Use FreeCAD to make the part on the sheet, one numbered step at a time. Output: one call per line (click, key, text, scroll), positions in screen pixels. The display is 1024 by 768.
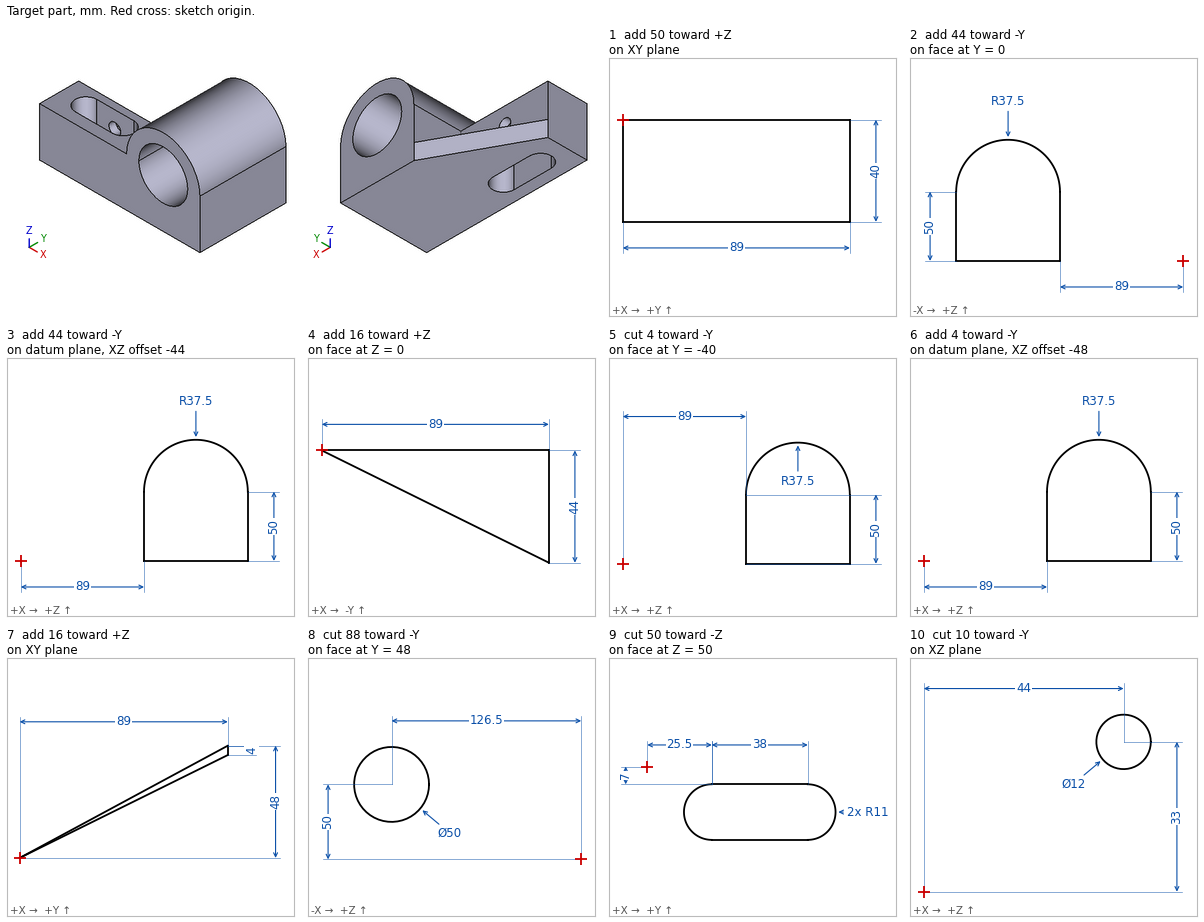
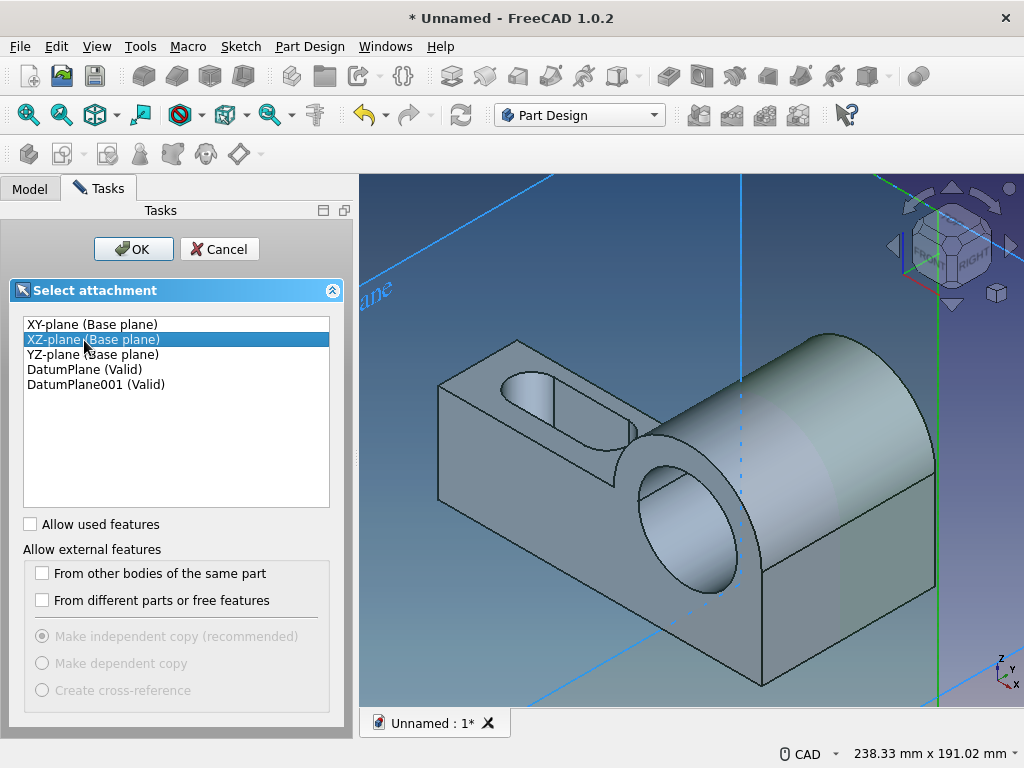
click(134, 249)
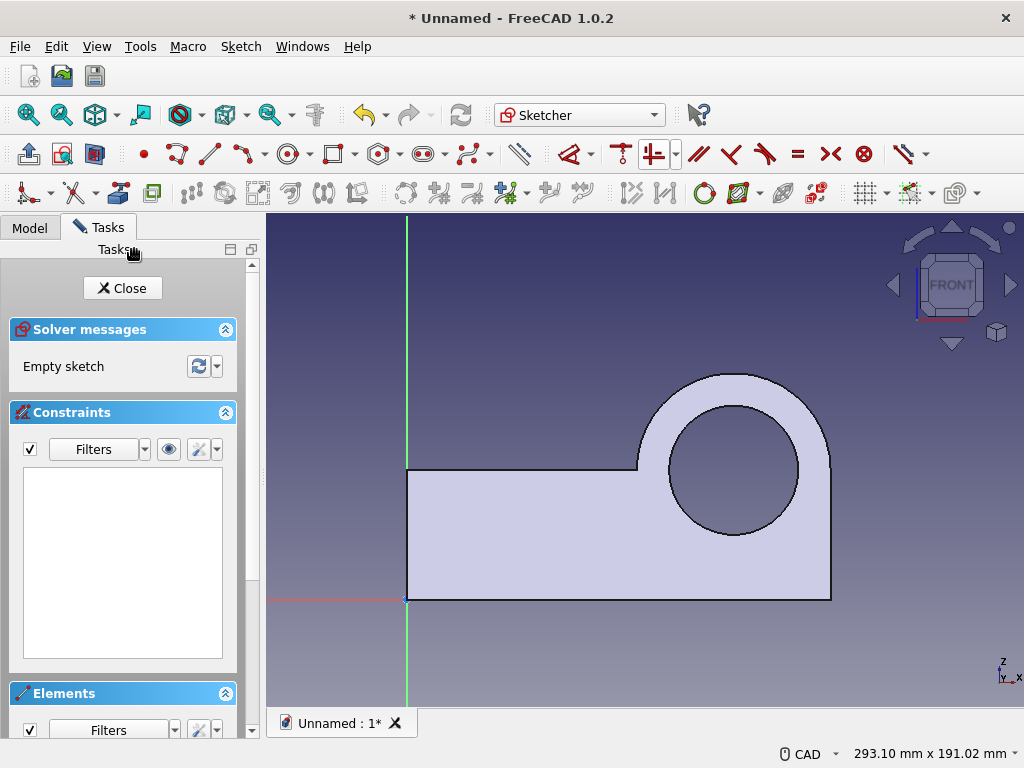
click(95, 154)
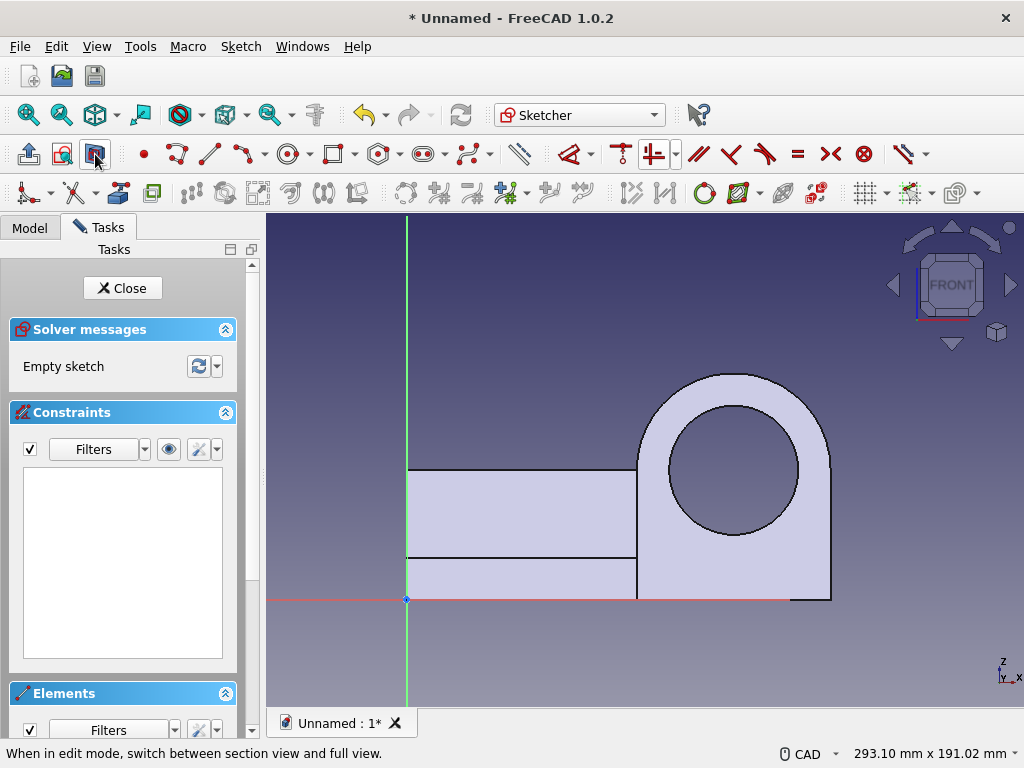
scroll(513, 521, up, 11)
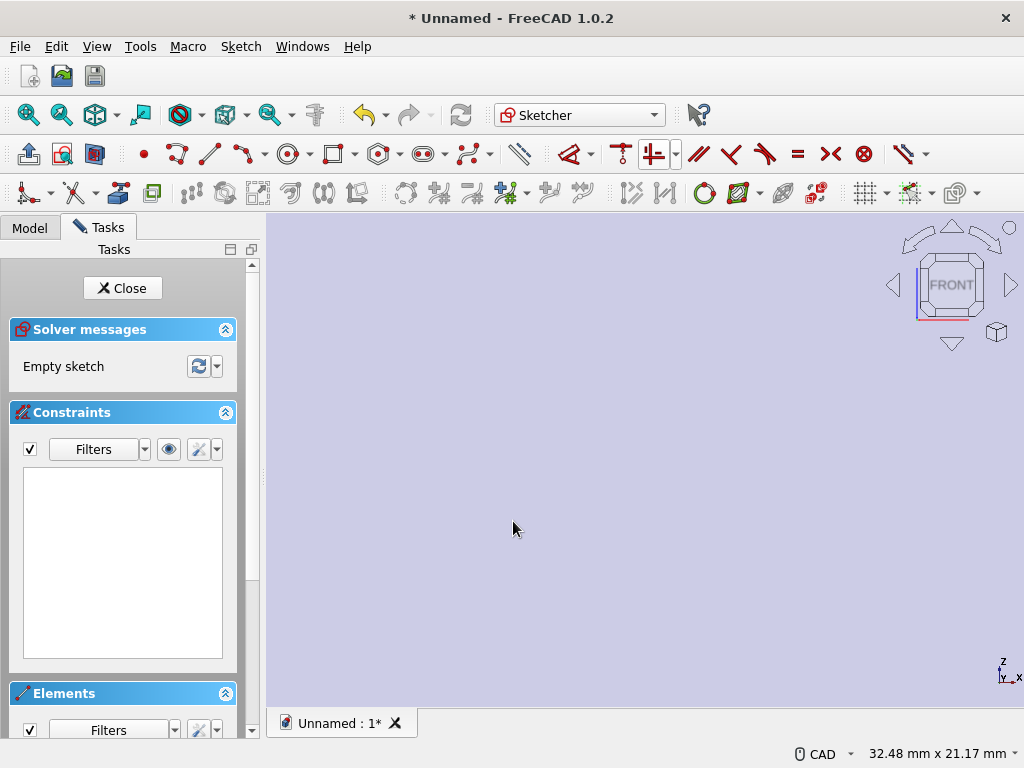
click(288, 154)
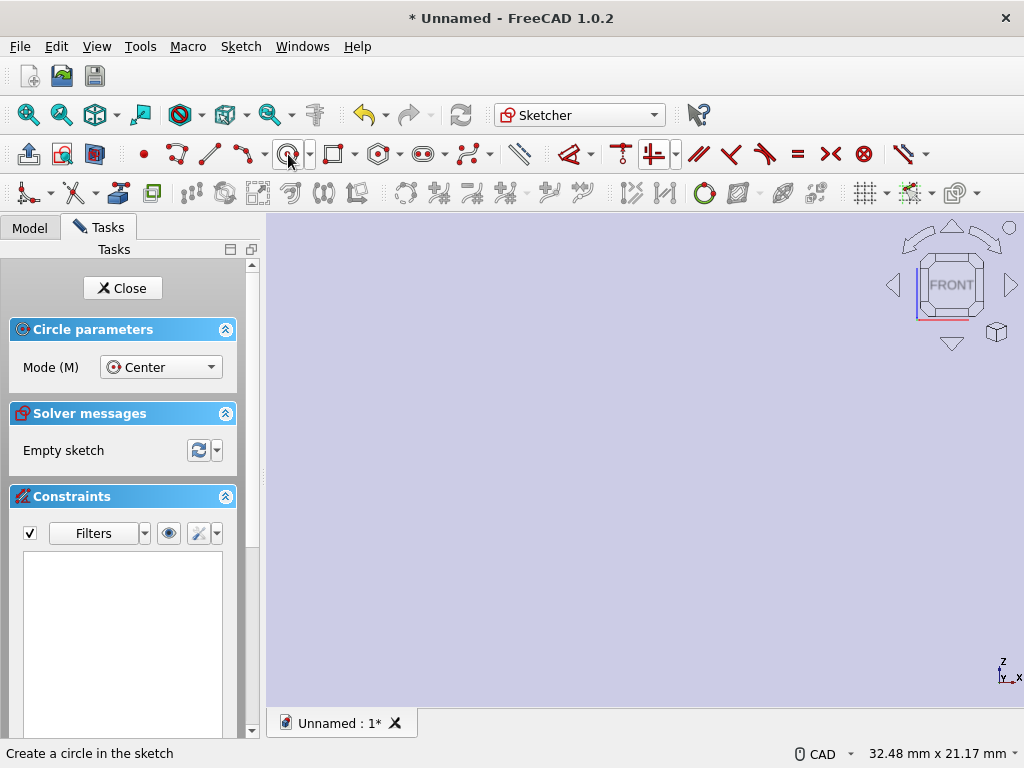
click(577, 454)
move(676, 355)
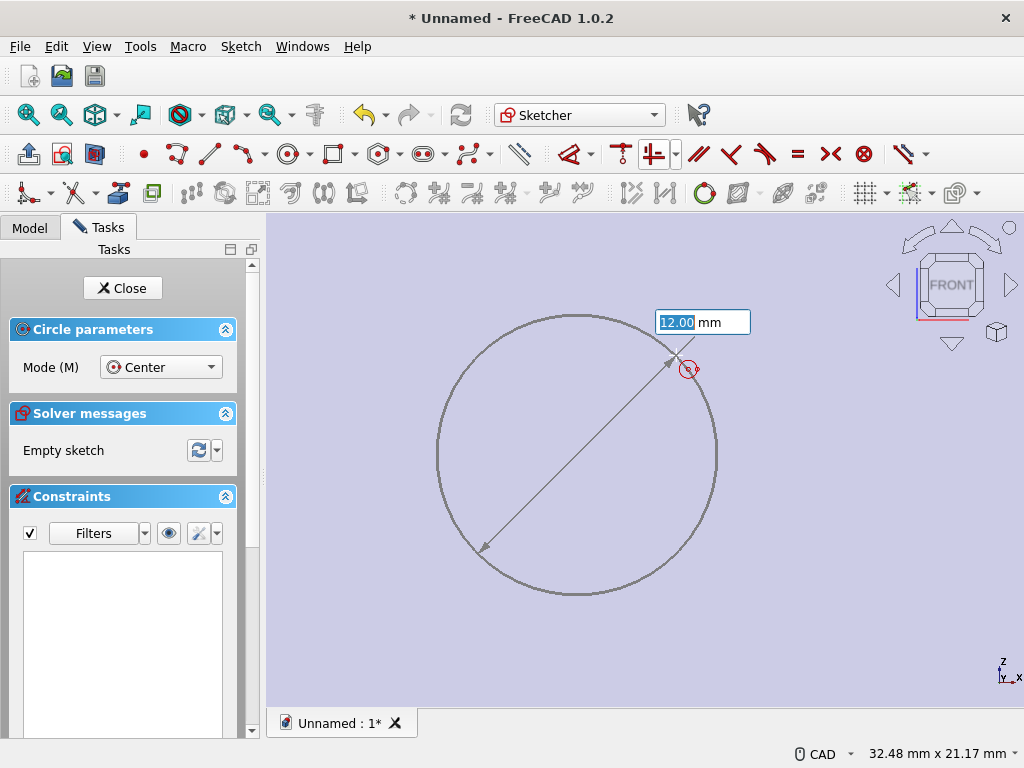
text(12)
key(Return)
key(Escape)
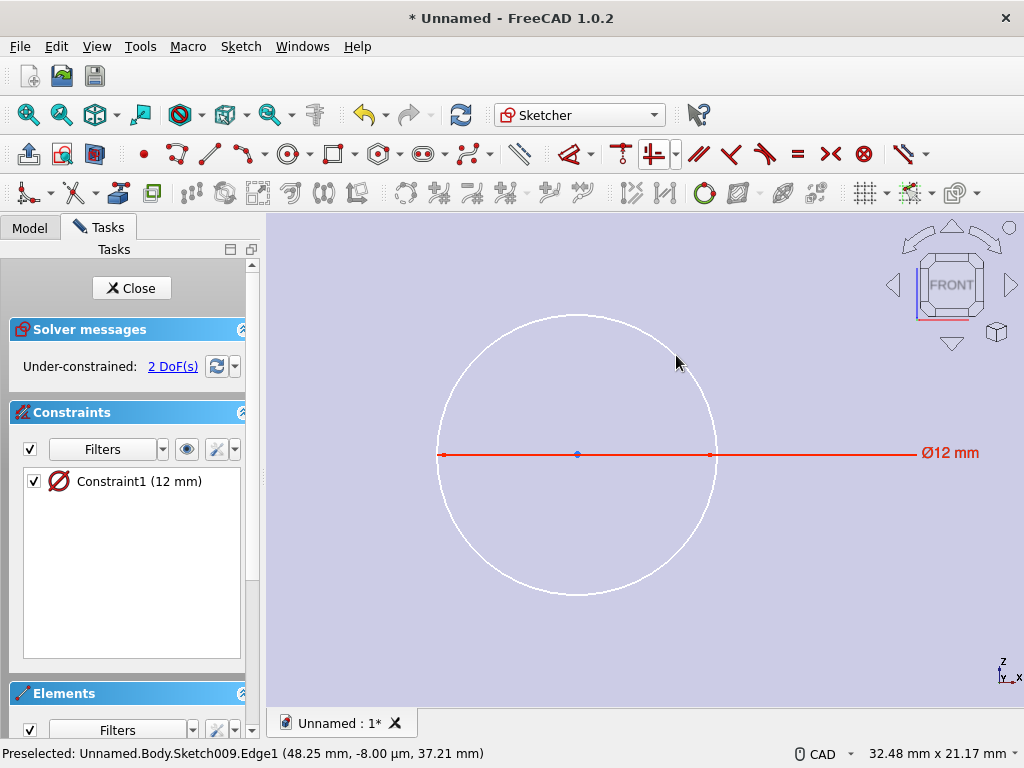
click(568, 154)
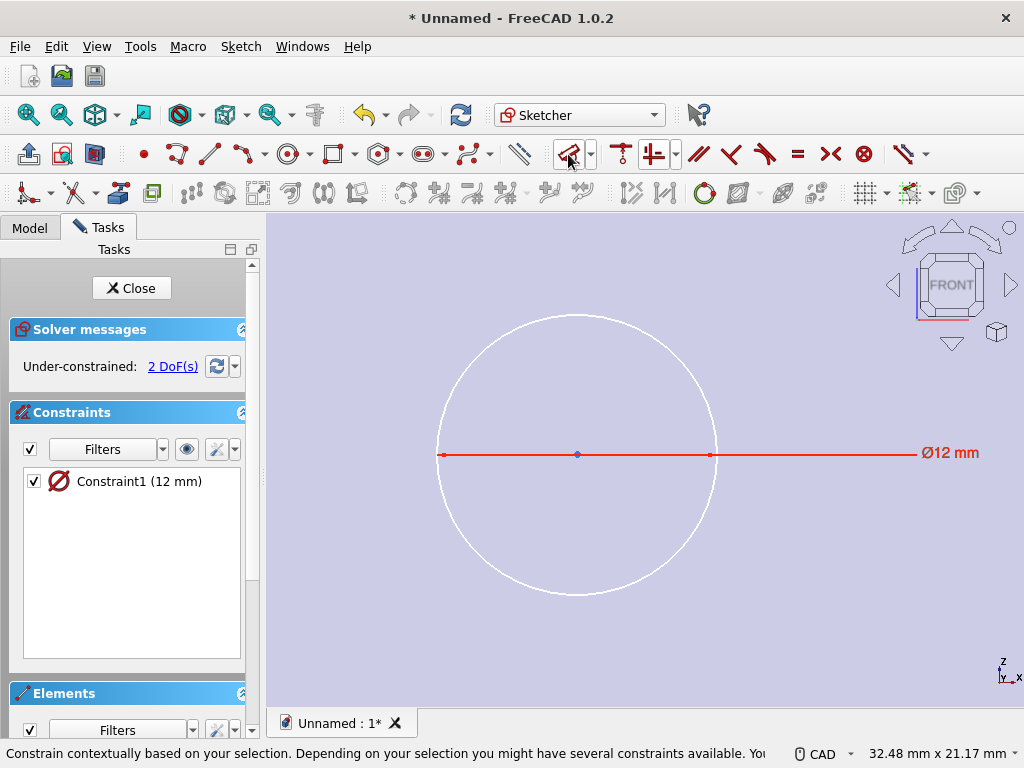
click(577, 455)
click(370, 421)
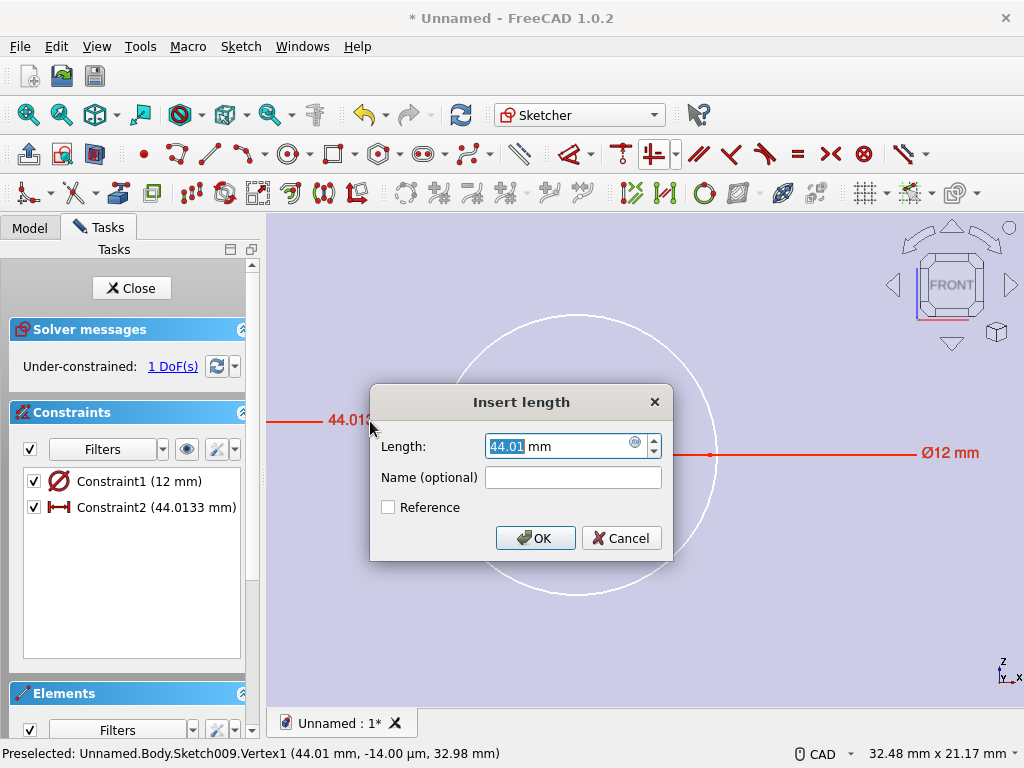
text(44)
key(Return)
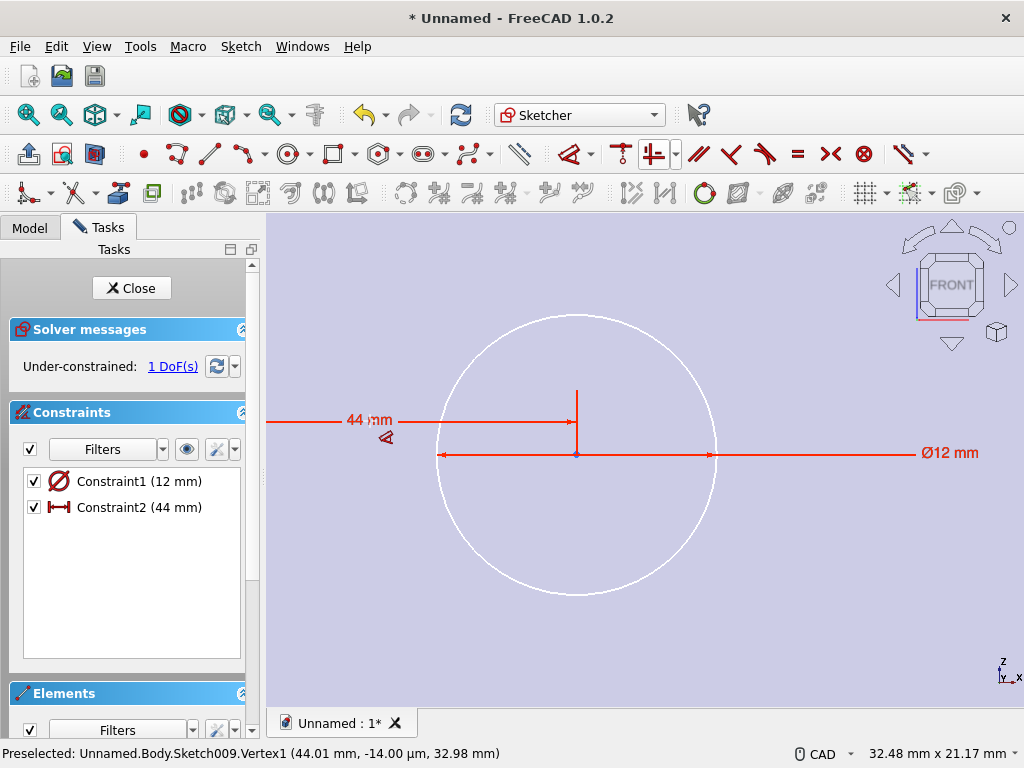
click(577, 455)
click(611, 567)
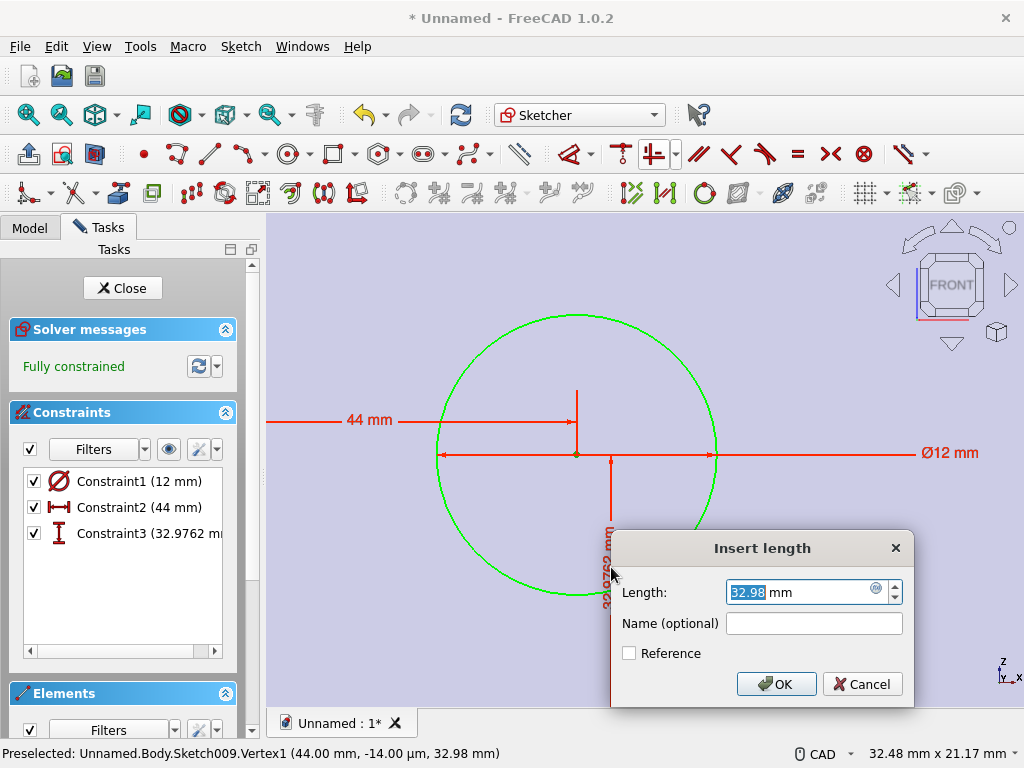
text(33)
key(Return)
key(Escape)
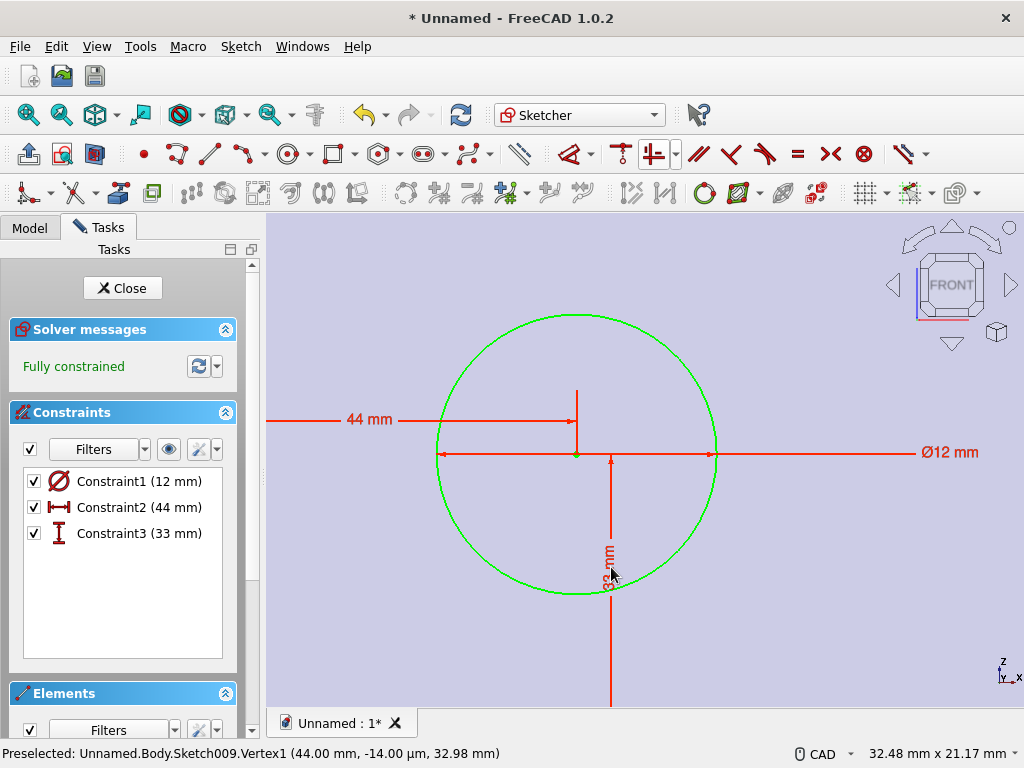
click(123, 288)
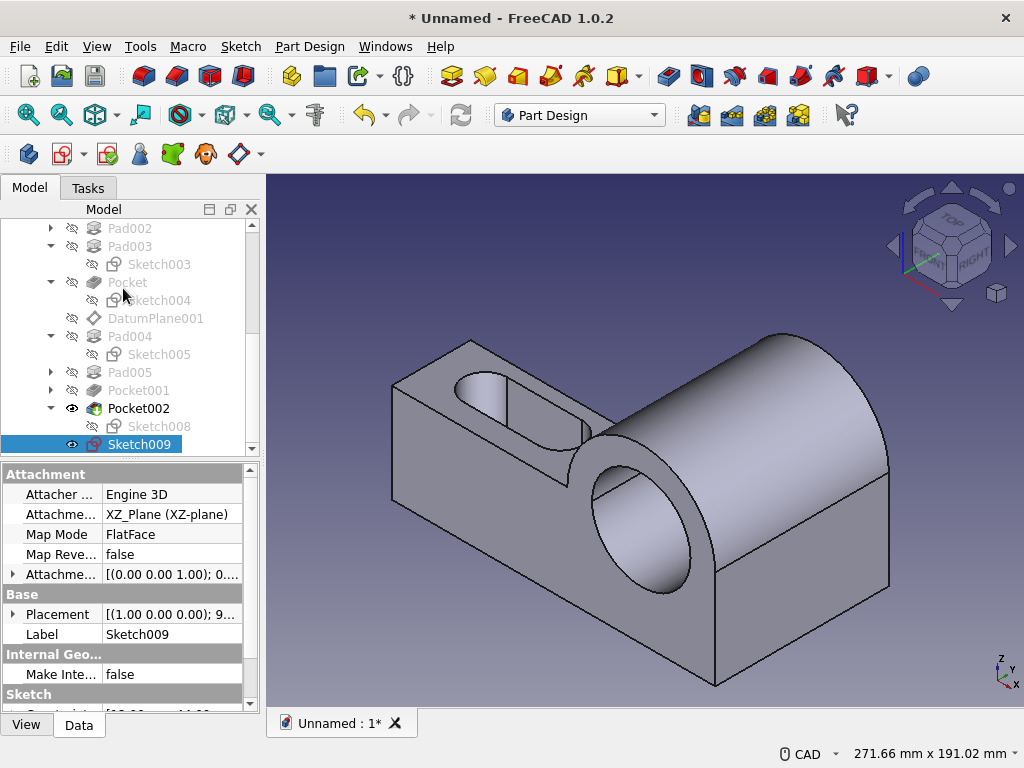
click(669, 76)